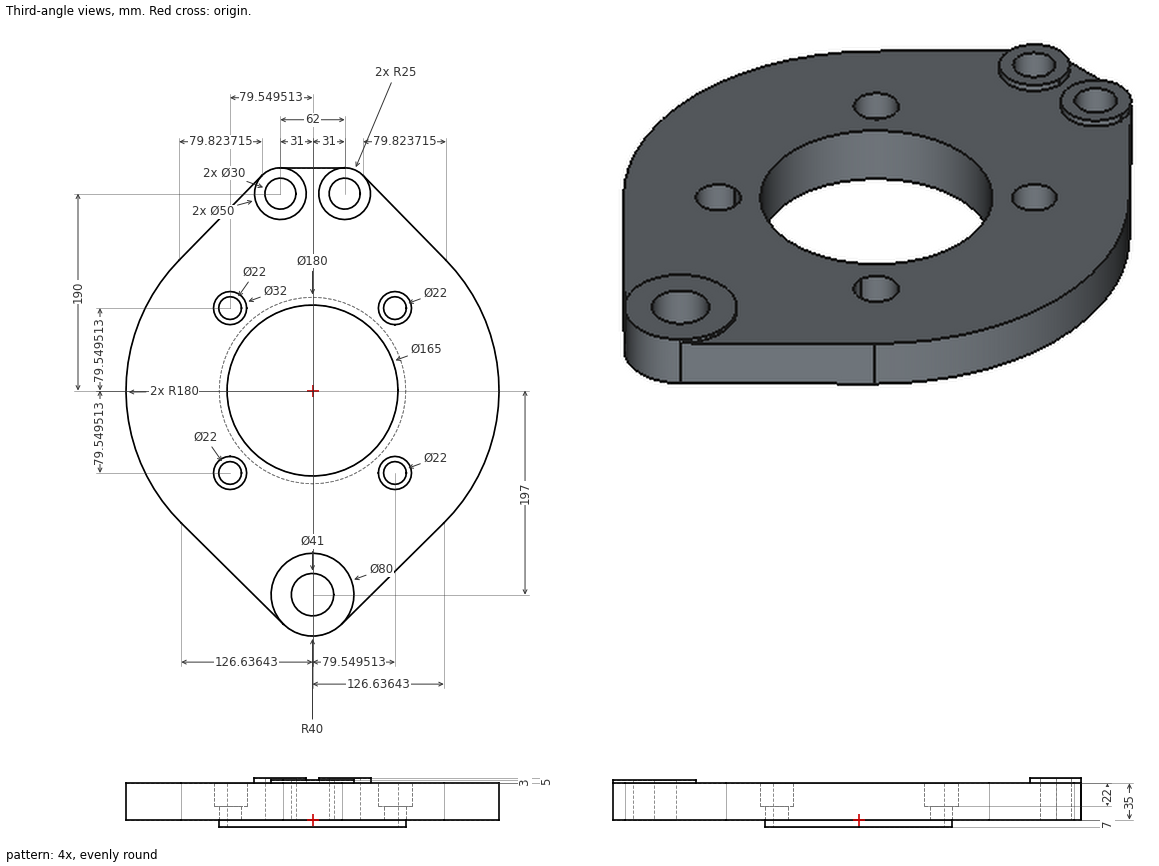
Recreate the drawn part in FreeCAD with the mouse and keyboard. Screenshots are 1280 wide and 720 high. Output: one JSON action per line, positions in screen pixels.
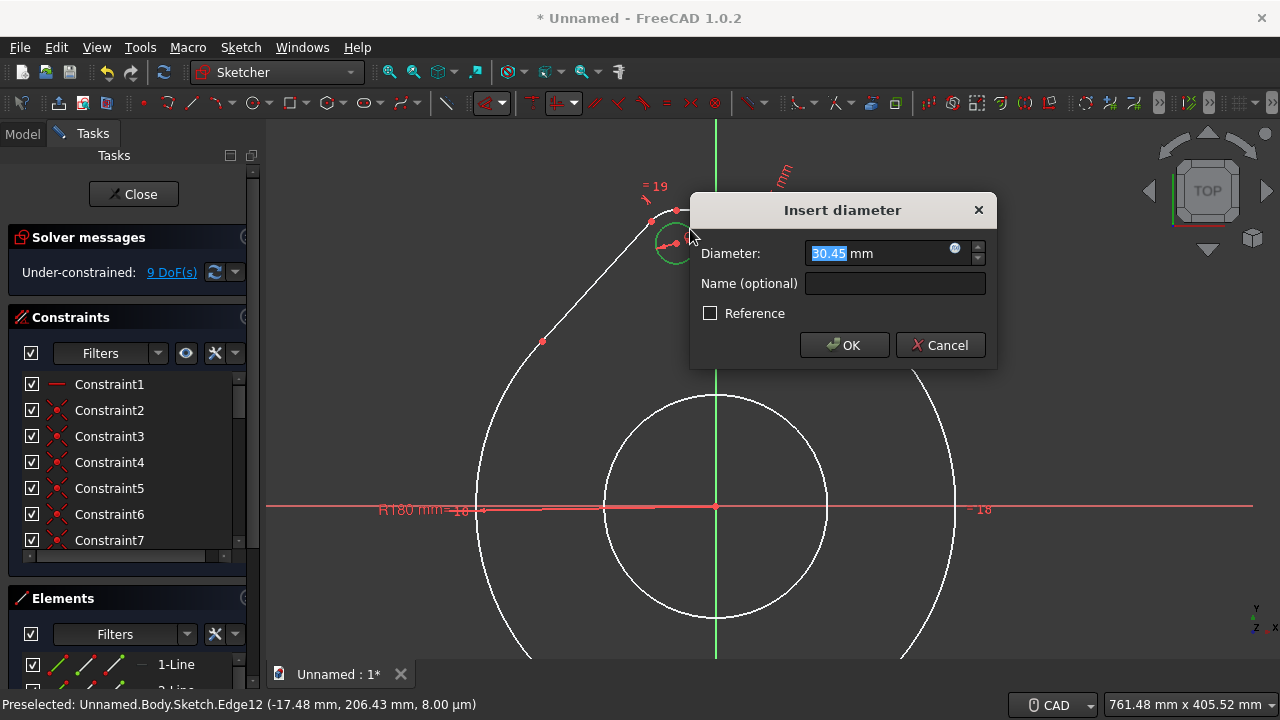
{"action": "type", "text": "30"}
{"action": "key", "text": "Return"}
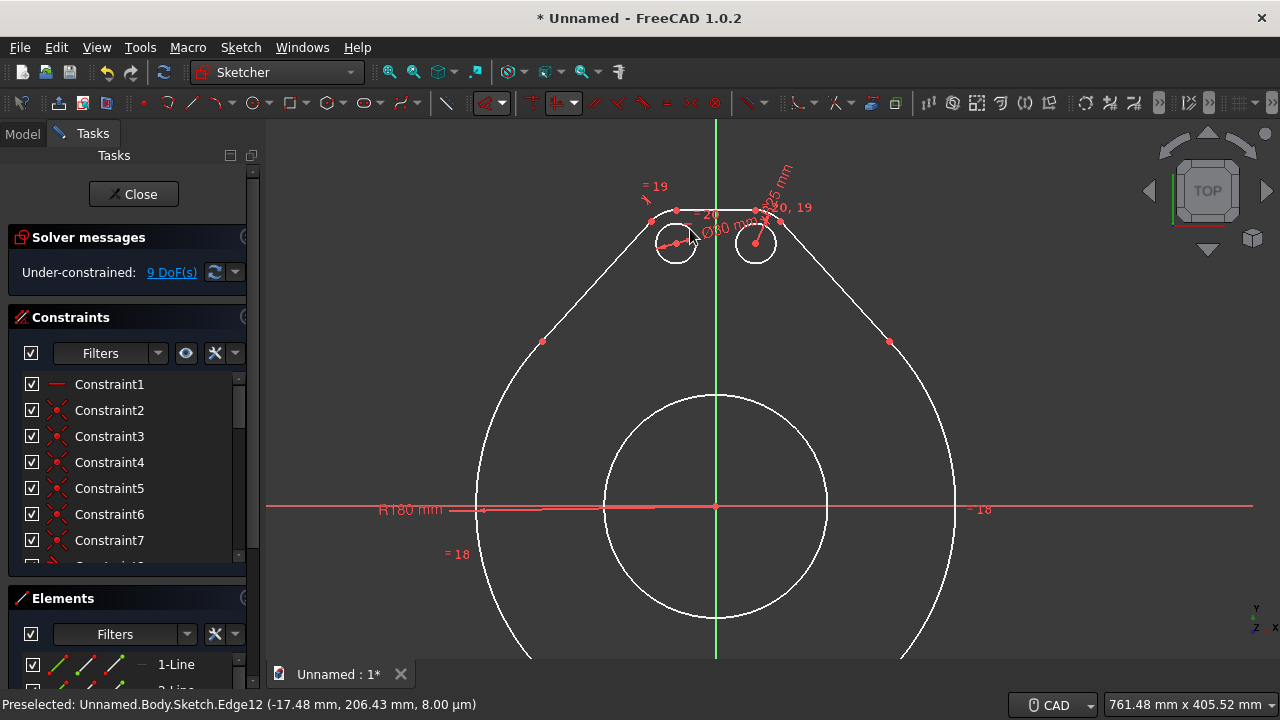
{"action": "left_click", "coordinate": [794, 427]}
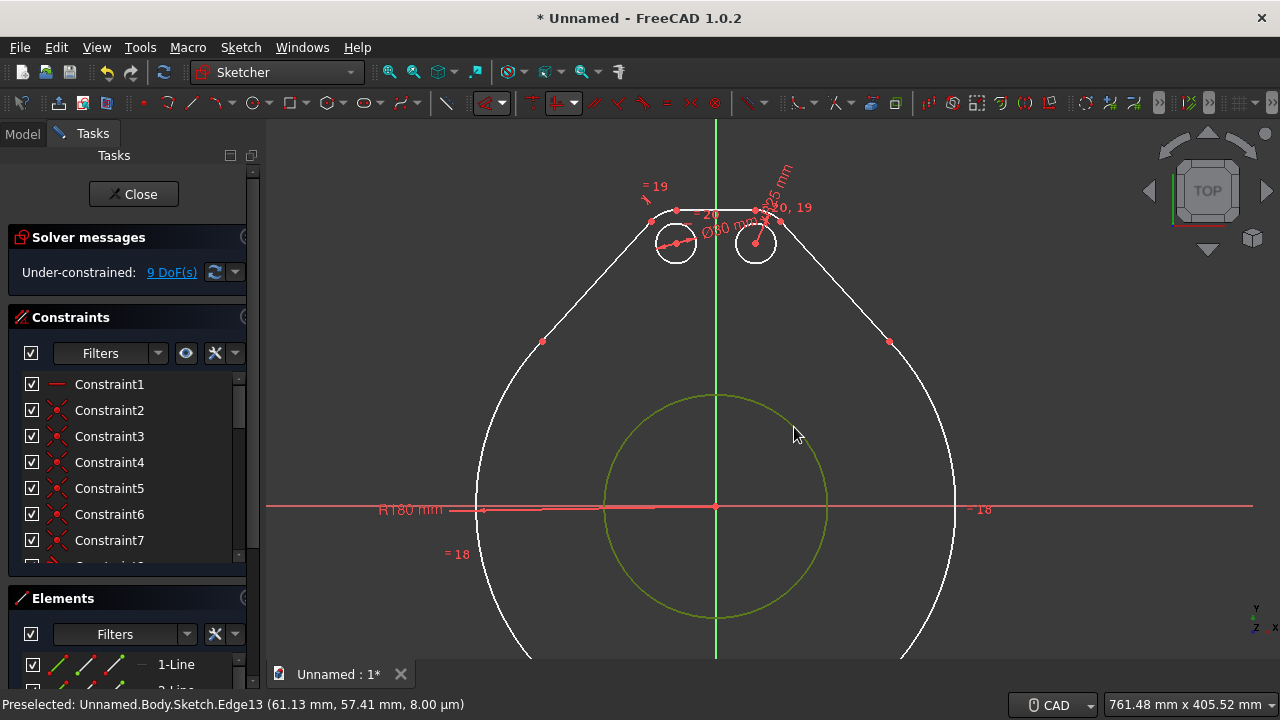
{"action": "key", "text": "k o"}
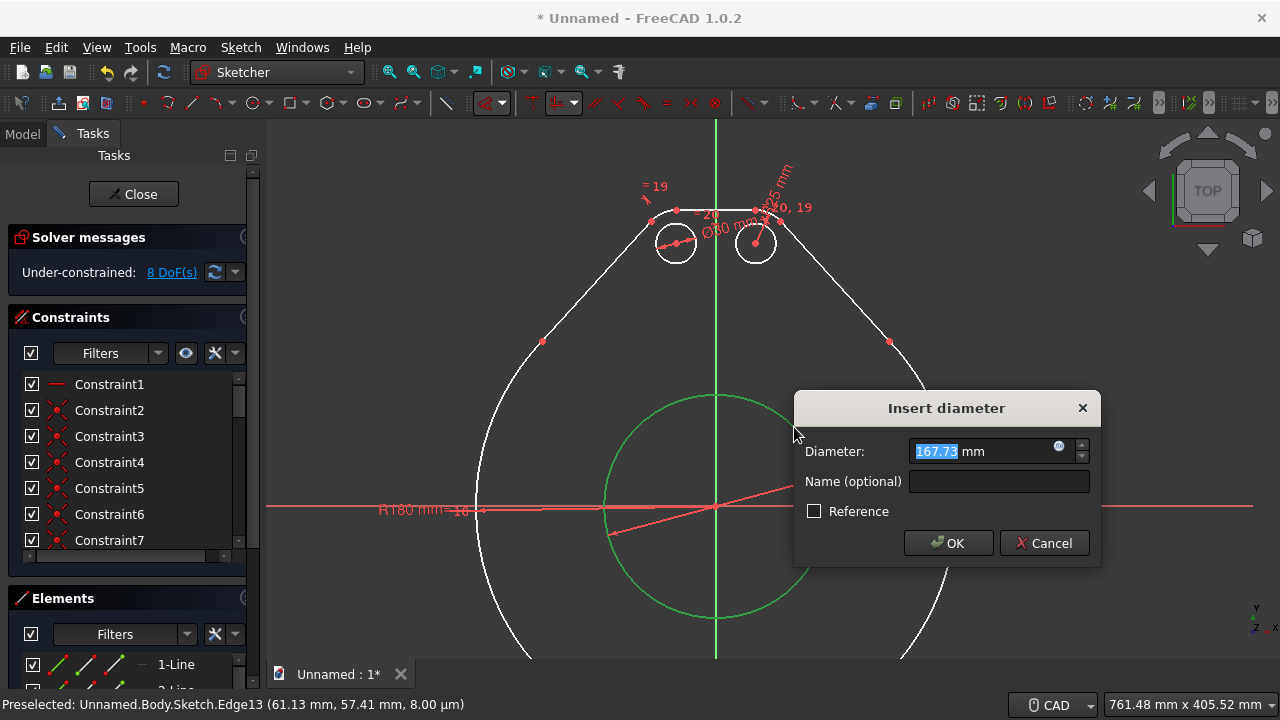
{"action": "type", "text": "165"}
{"action": "key", "text": "Return"}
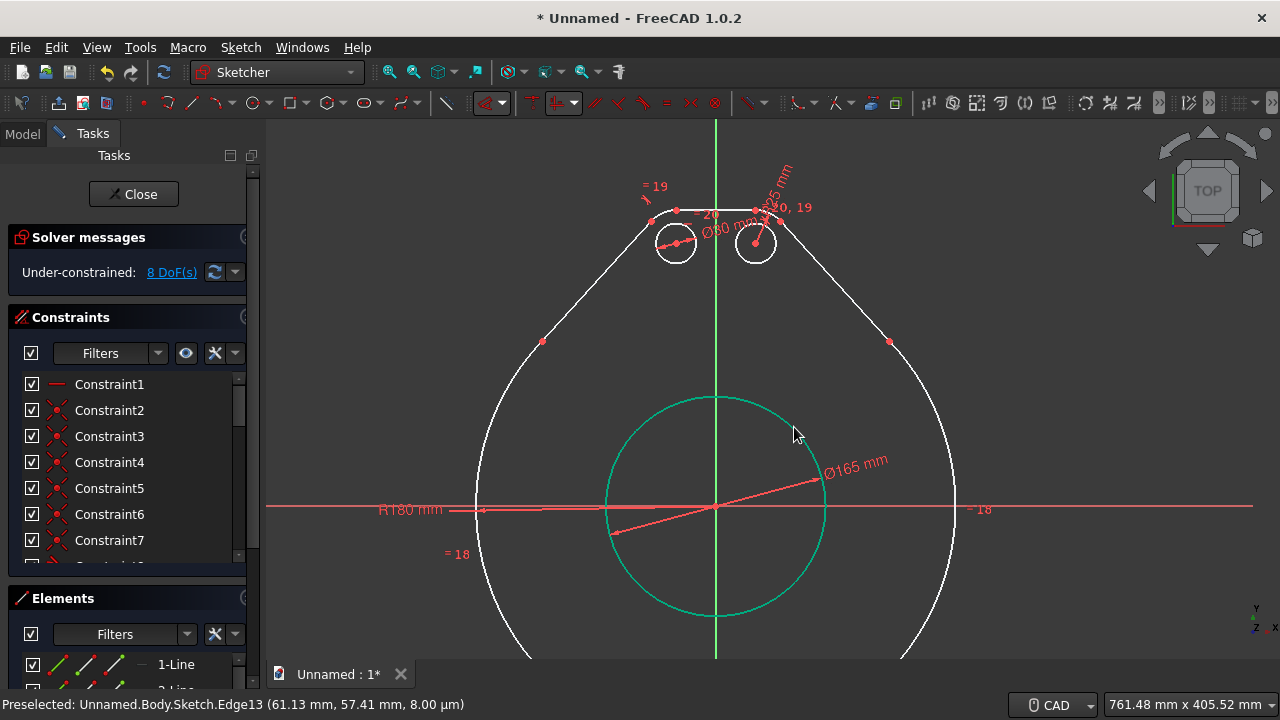
{"action": "left_click", "coordinate": [732, 210]}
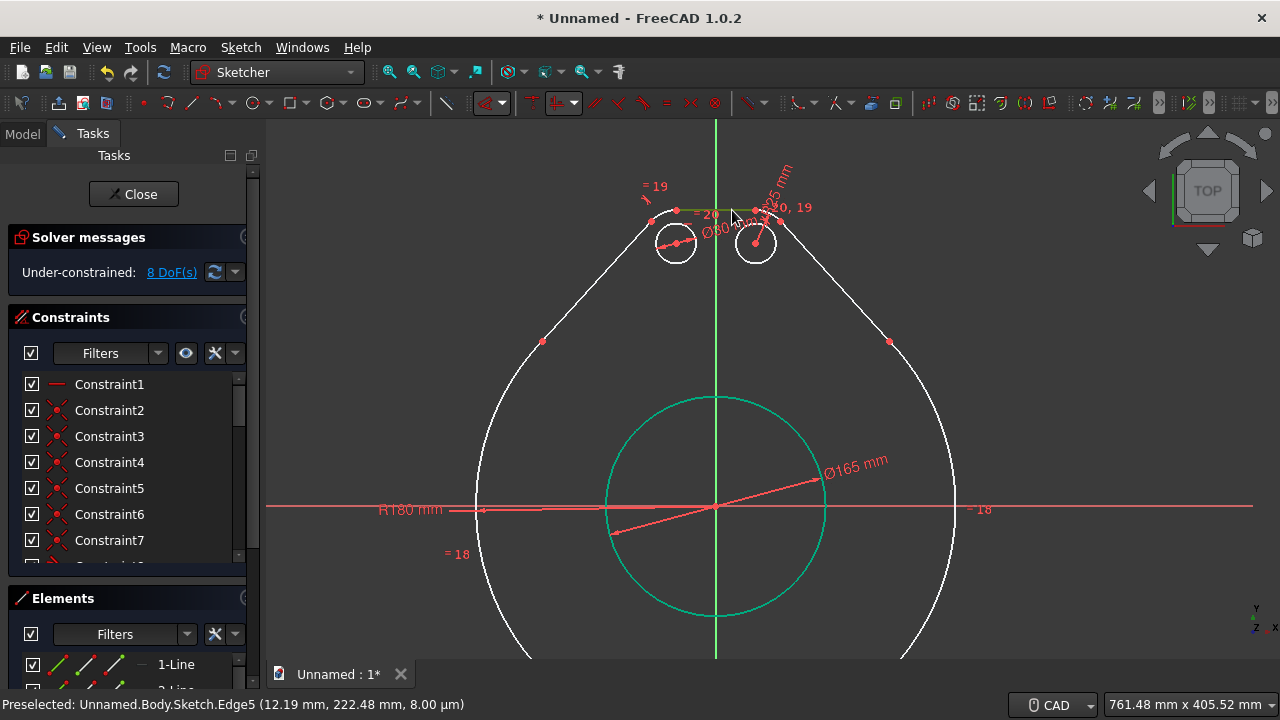
{"action": "key", "text": "l"}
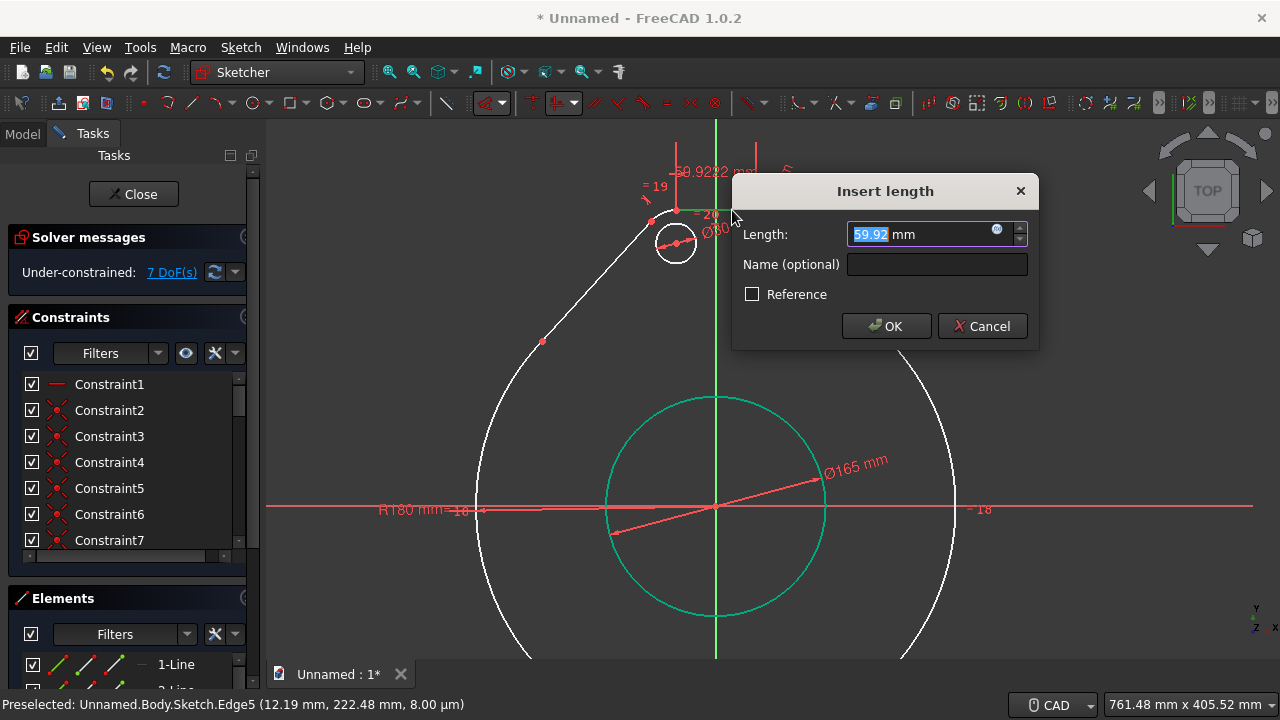
{"action": "type", "text": "62"}
{"action": "key", "text": "Return"}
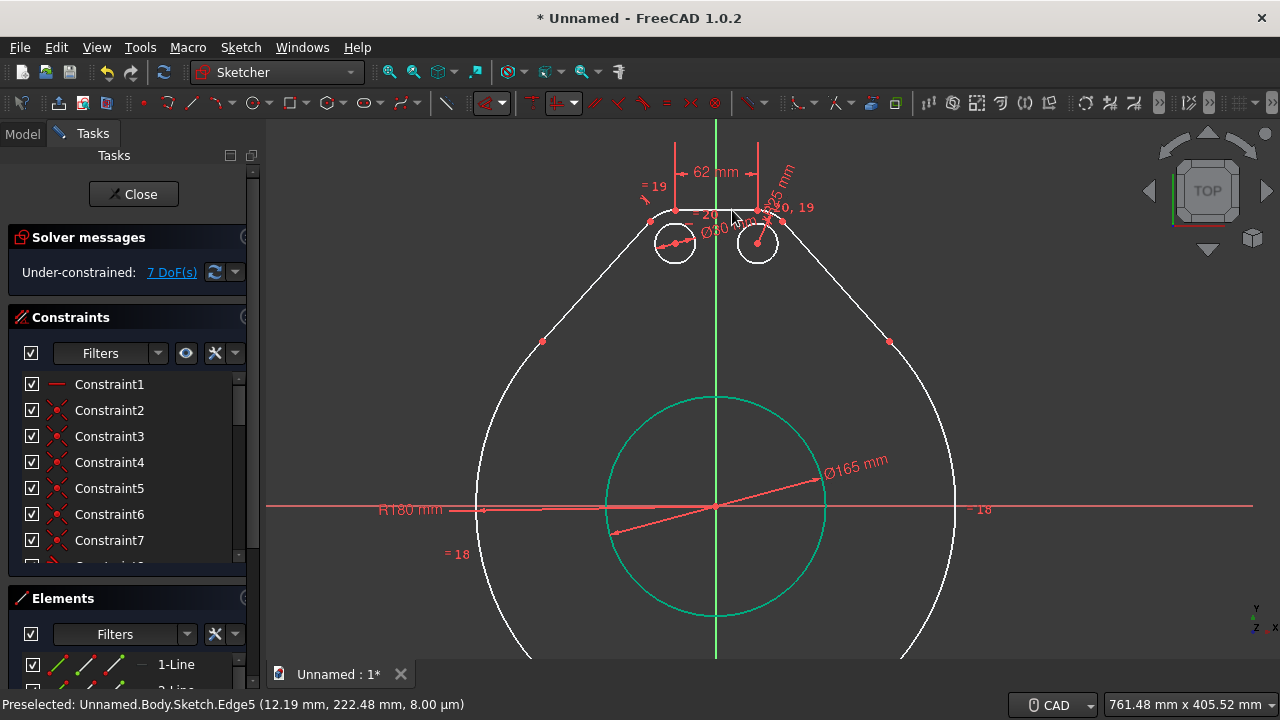
{"action": "left_click", "coordinate": [675, 243]}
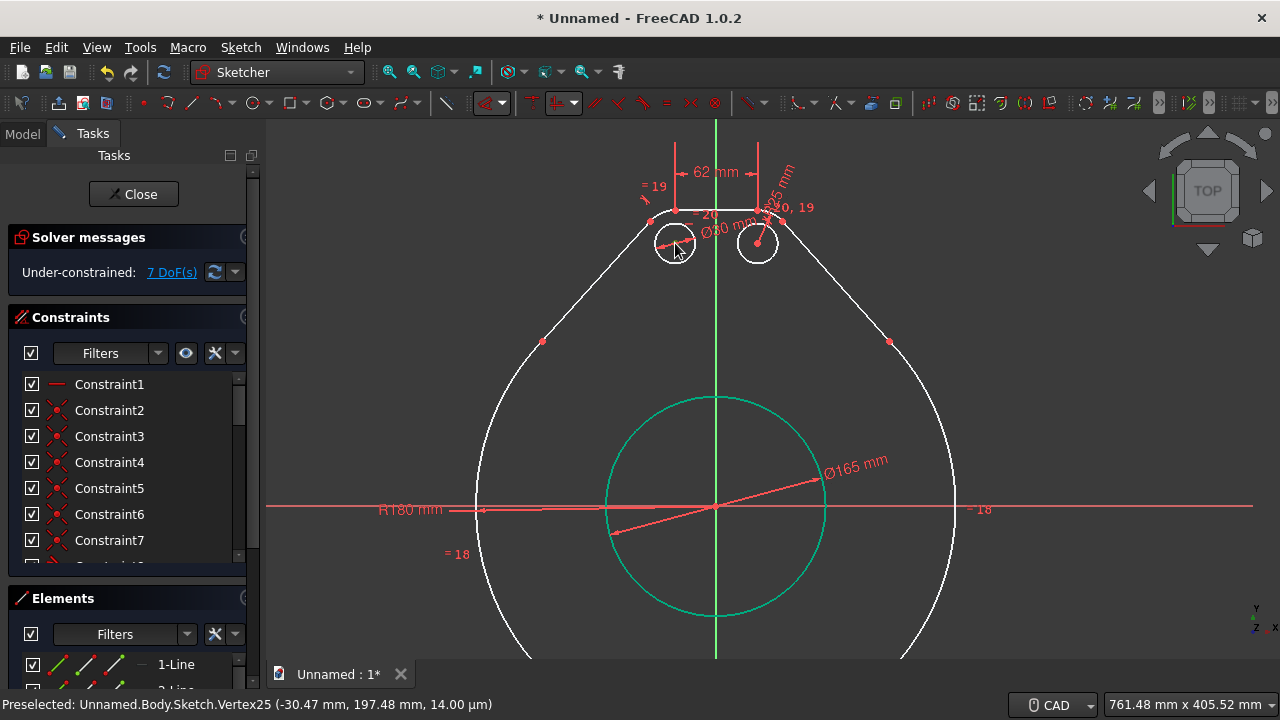
{"action": "key", "text": "l"}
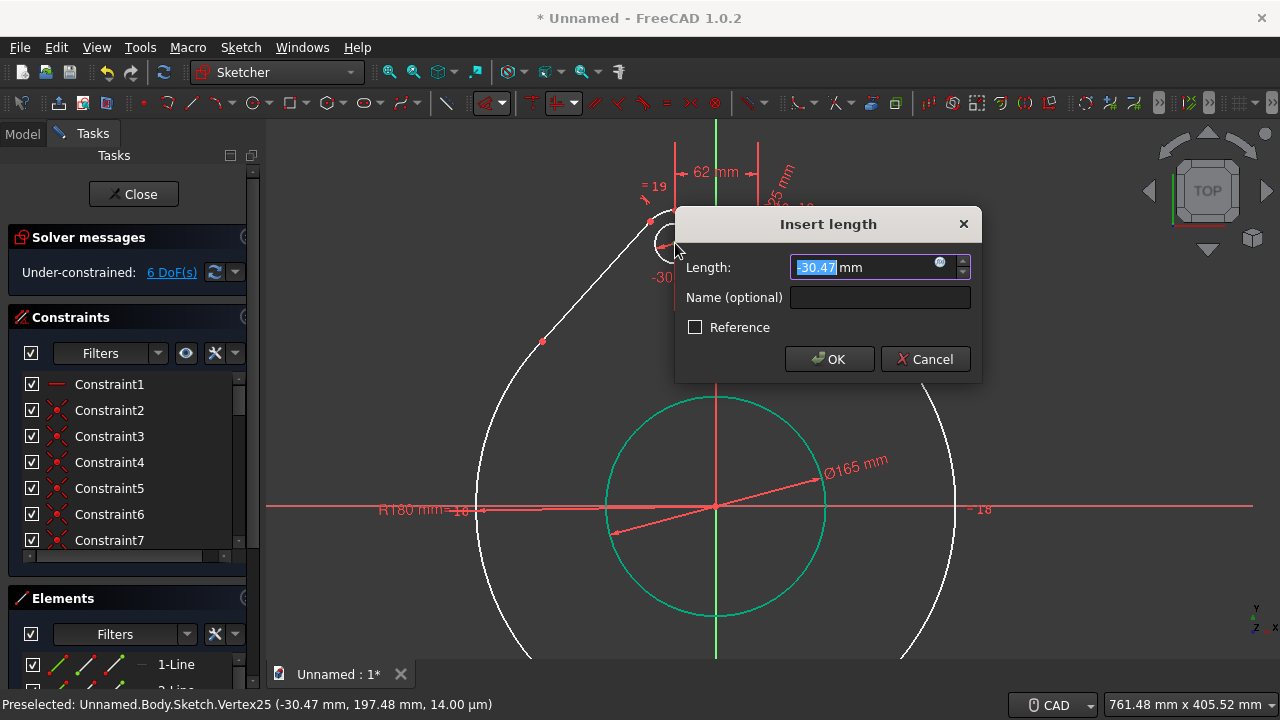
{"action": "type", "text": "-31"}
{"action": "key", "text": "Return"}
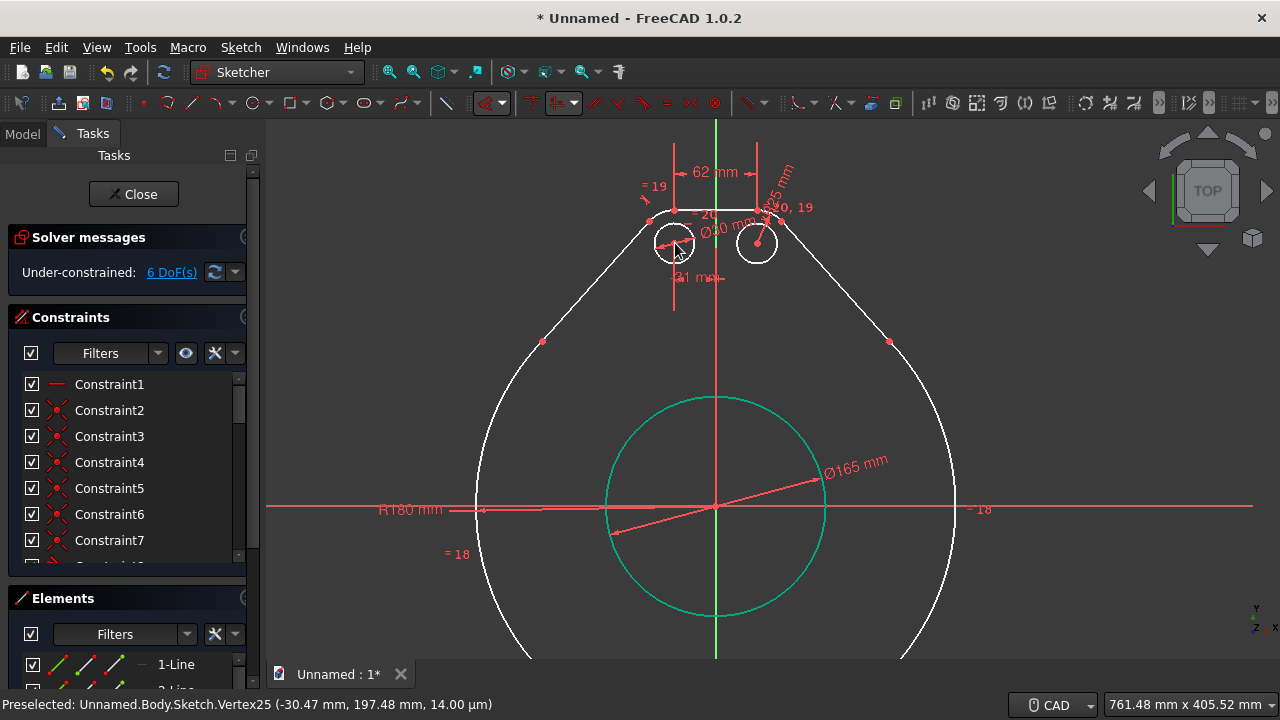
{"action": "scroll", "coordinate": [691, 228], "scroll_direction": "down", "scroll_amount": 3}